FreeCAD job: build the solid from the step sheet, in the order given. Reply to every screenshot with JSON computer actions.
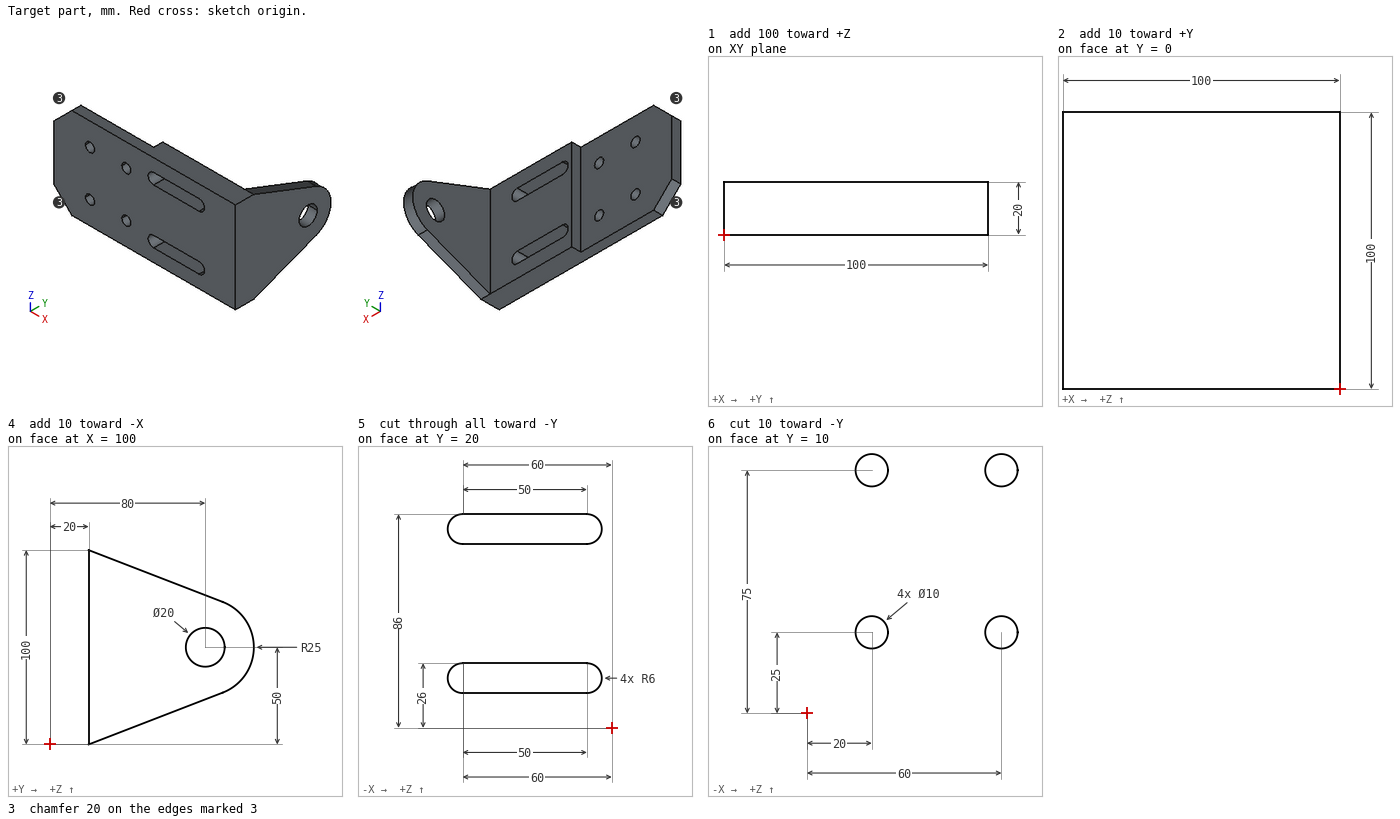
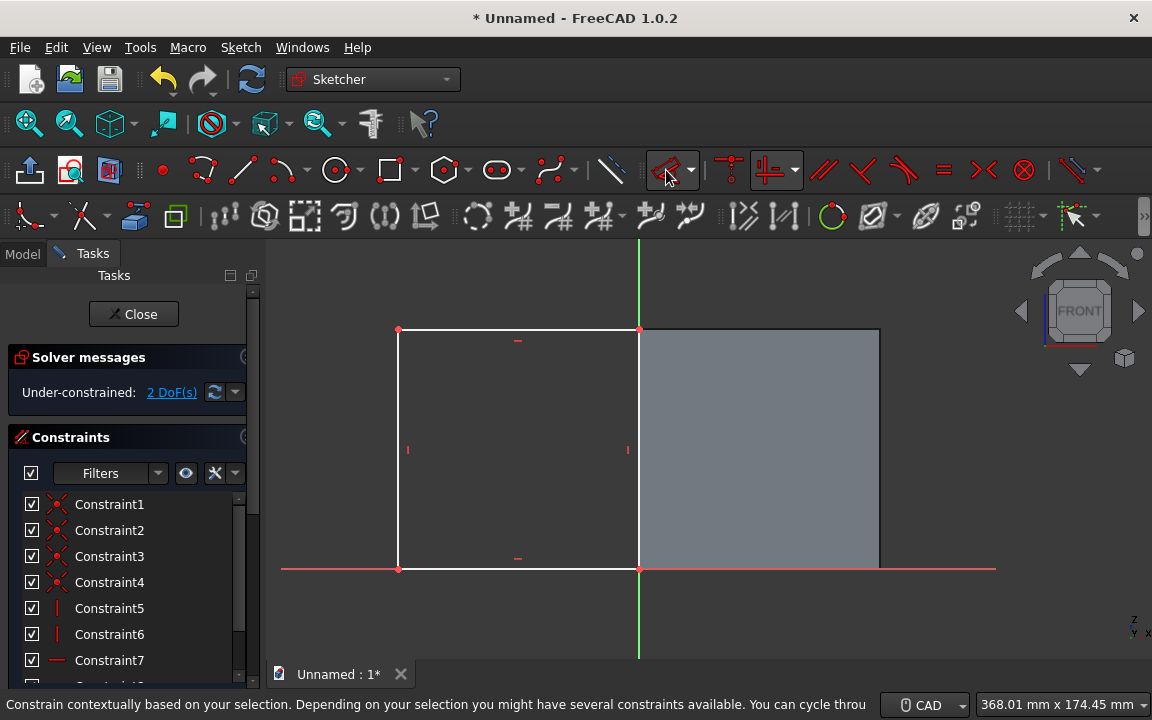
{"action": "left_click", "coordinate": [639, 498]}
{"action": "left_click", "coordinate": [673, 450]}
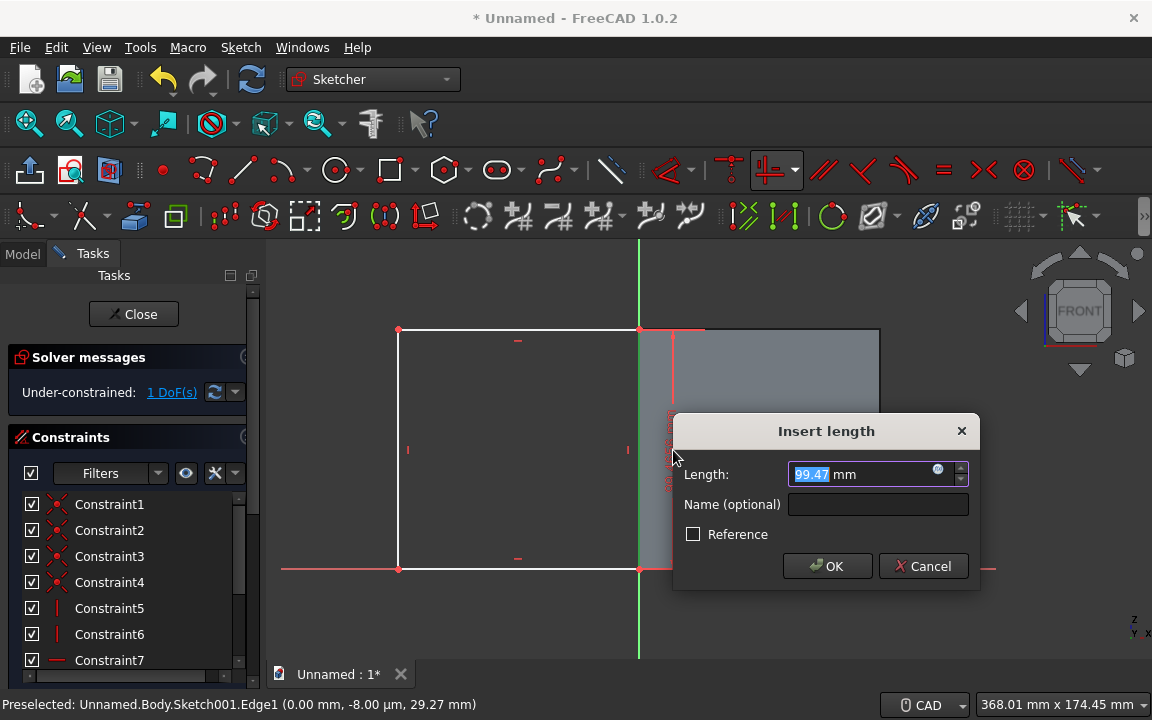
{"action": "type", "text": "100"}
{"action": "key", "text": "Return"}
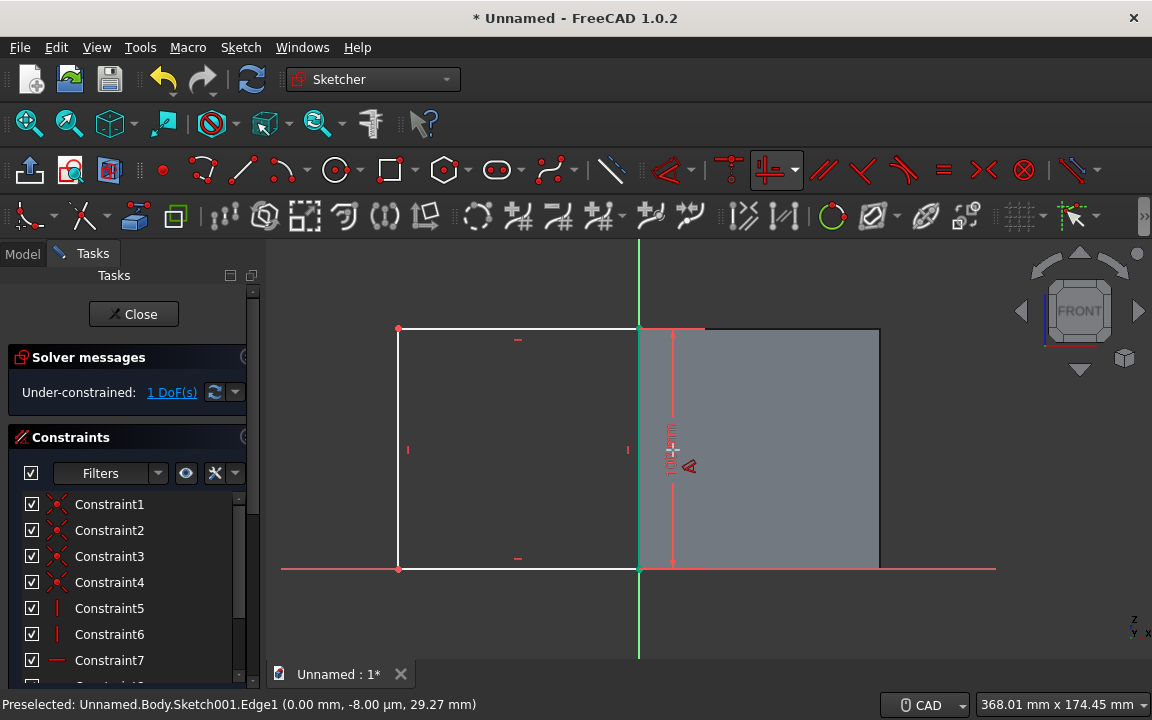
{"action": "left_click", "coordinate": [567, 329]}
{"action": "left_click", "coordinate": [519, 295]}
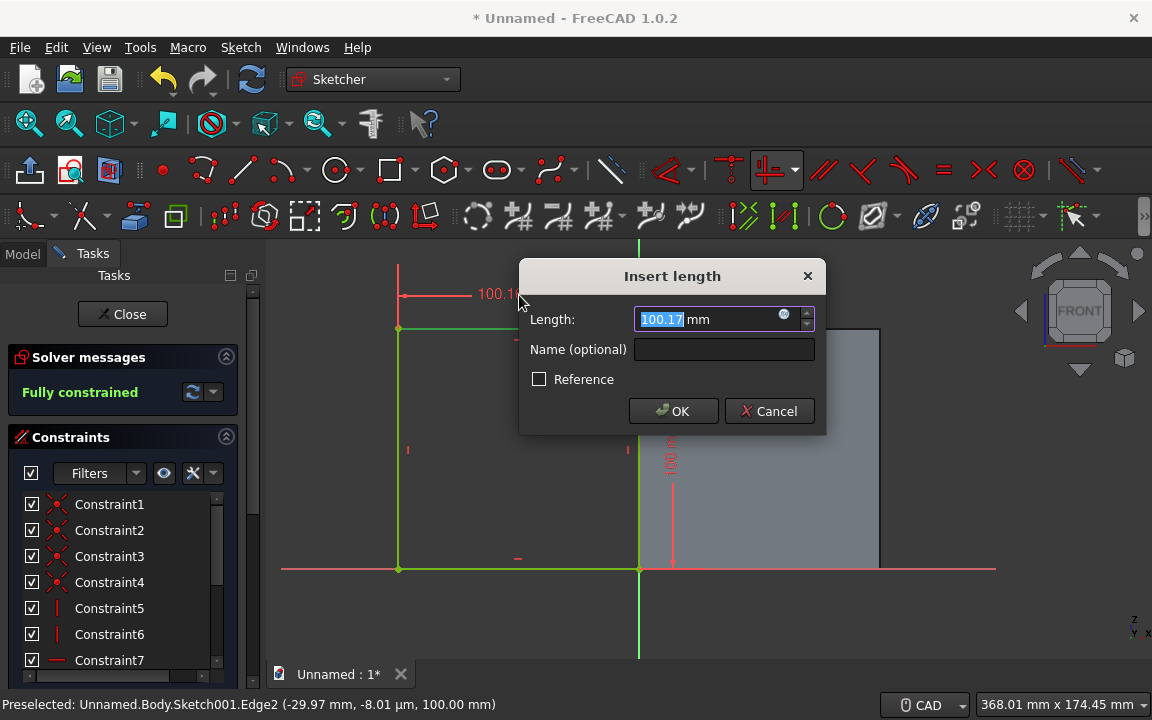
{"action": "type", "text": "100"}
{"action": "key", "text": "Return"}
{"action": "key", "text": "Escape"}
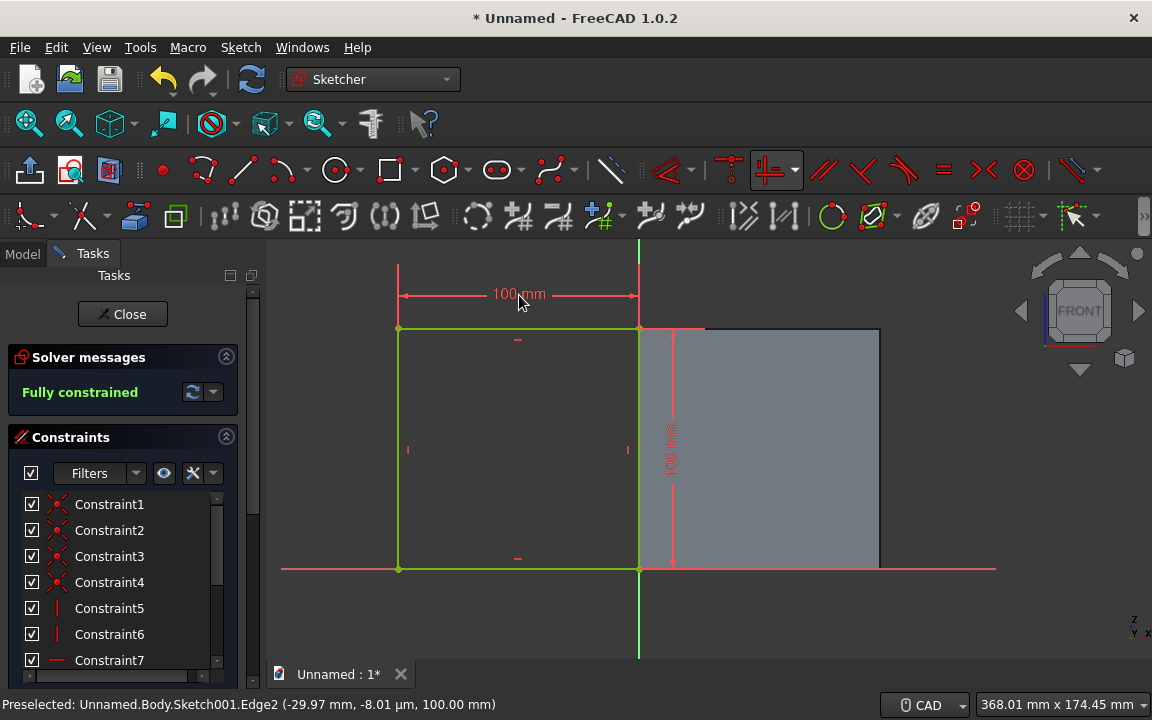
{"action": "left_click", "coordinate": [123, 314]}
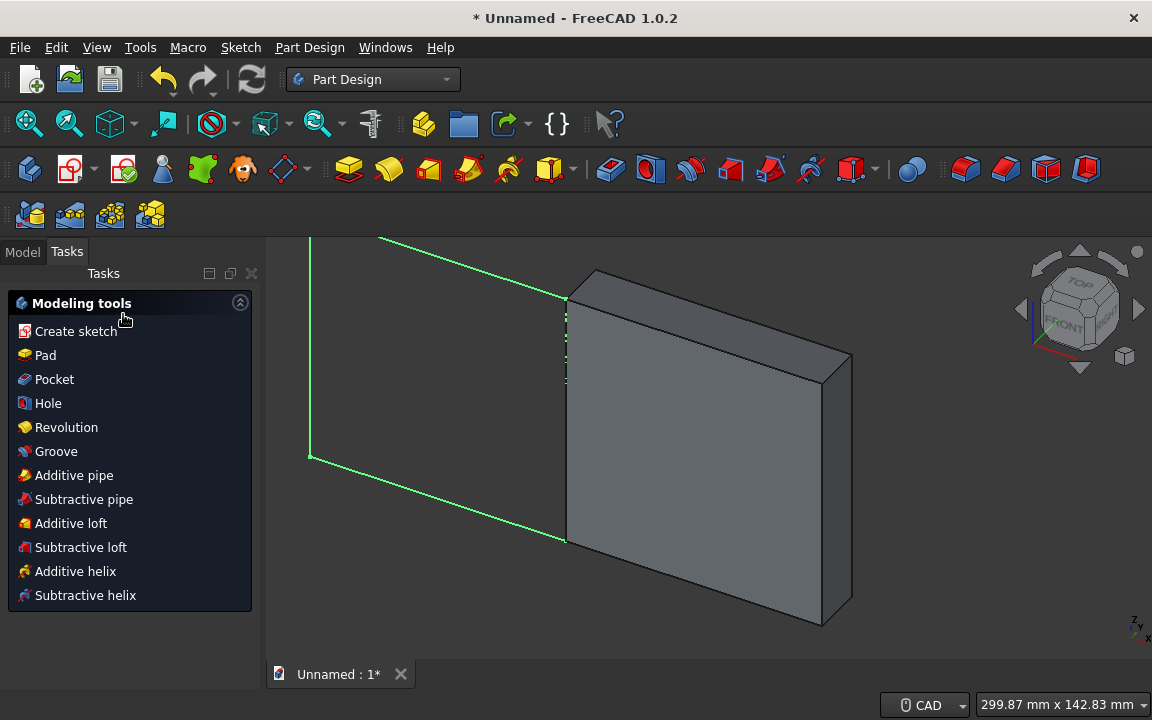
{"action": "left_click", "coordinate": [350, 170]}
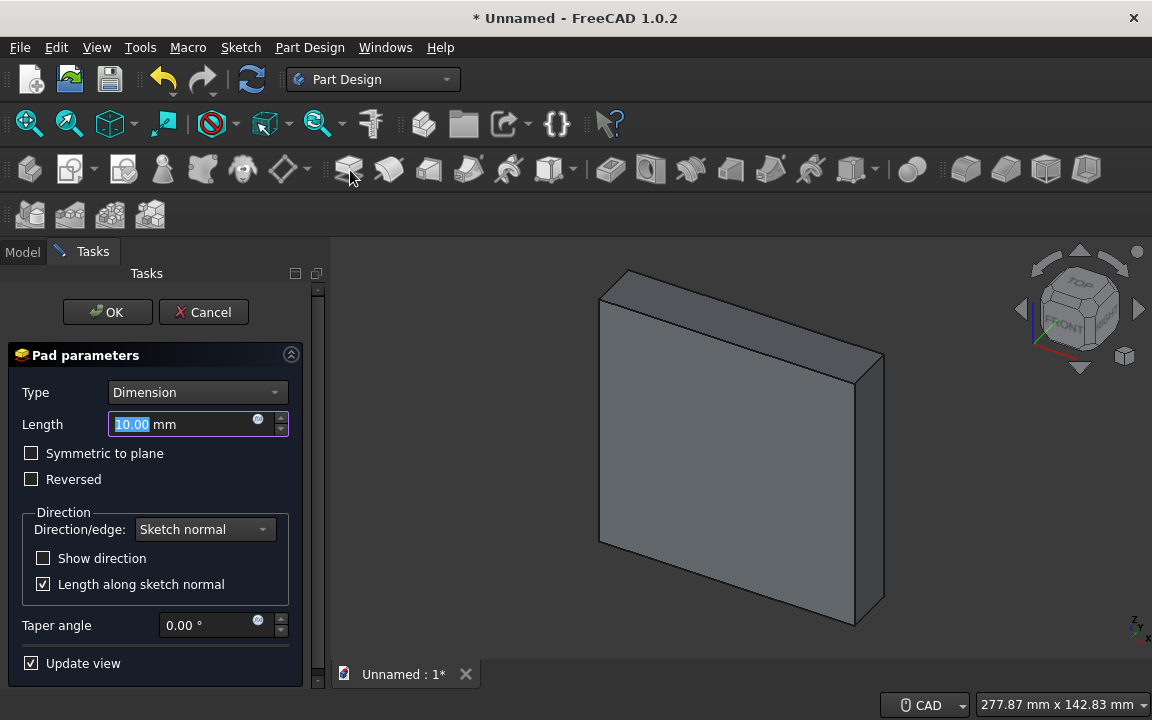
{"action": "type", "text": "10"}
{"action": "key", "text": "Tab"}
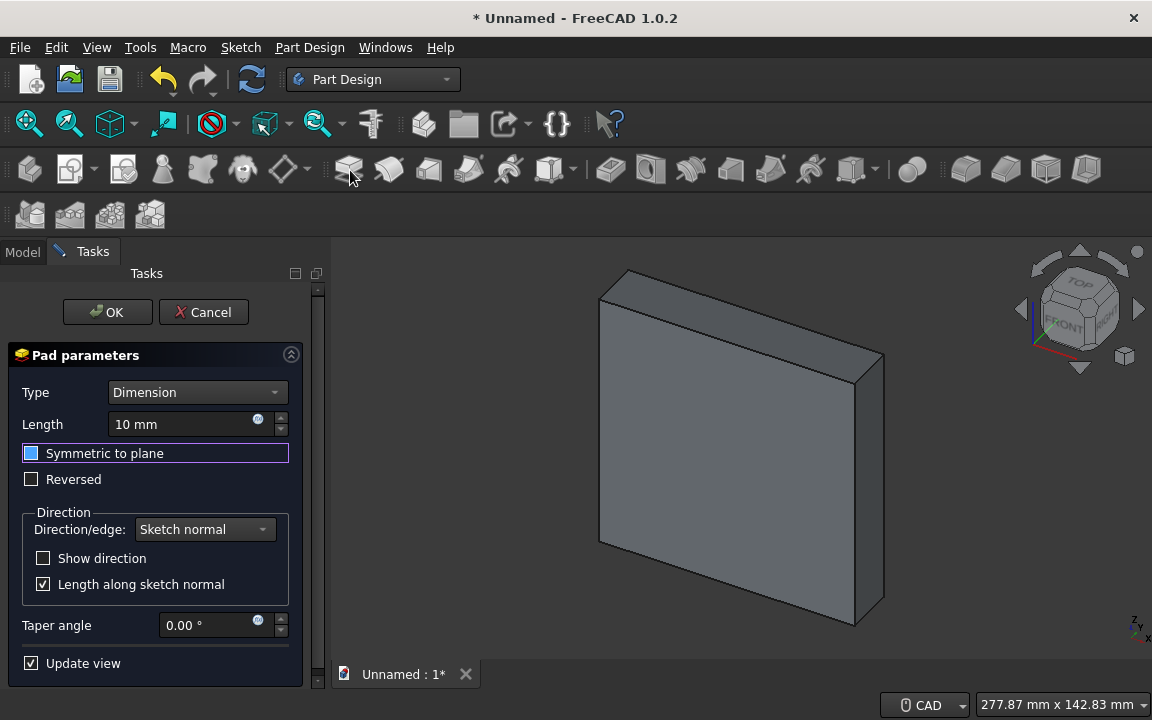
{"action": "left_click", "coordinate": [30, 479]}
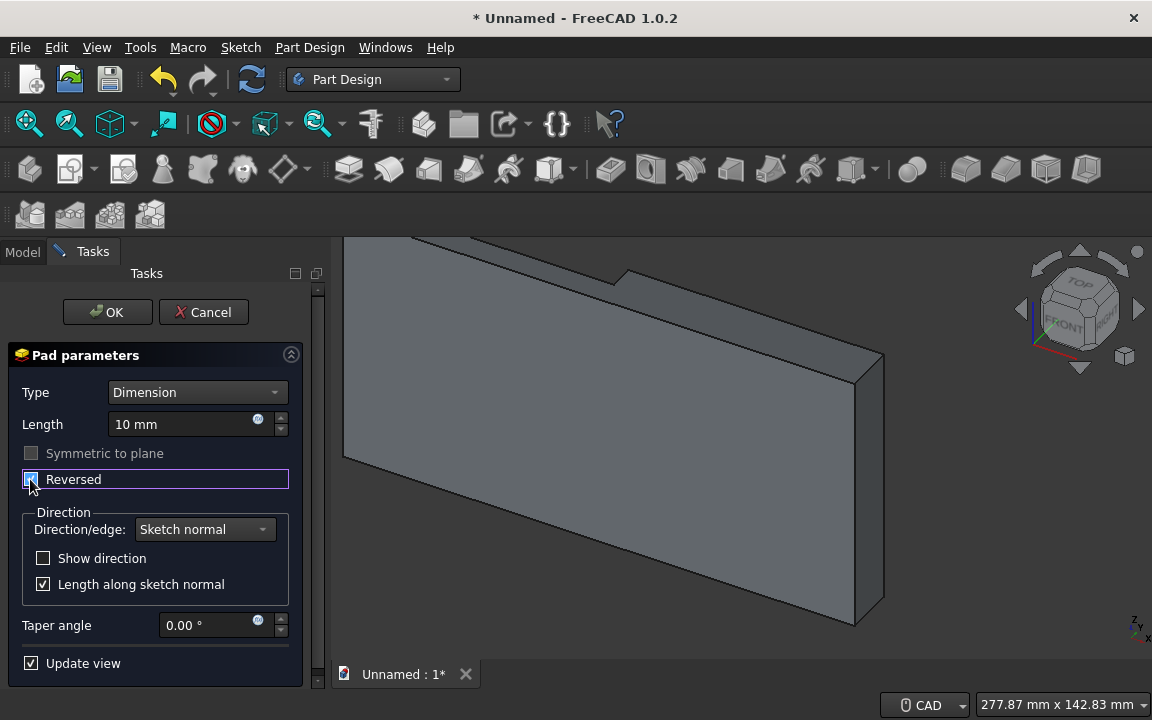
{"action": "left_click", "coordinate": [108, 312]}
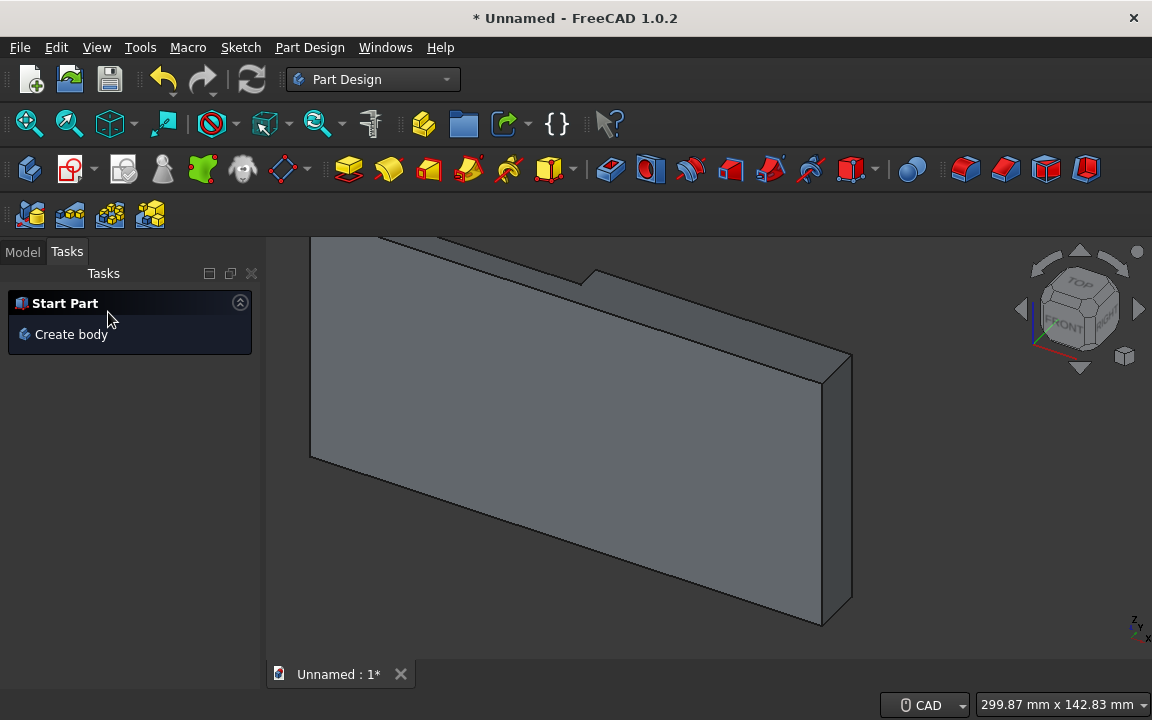
{"action": "left_click", "coordinate": [30, 124]}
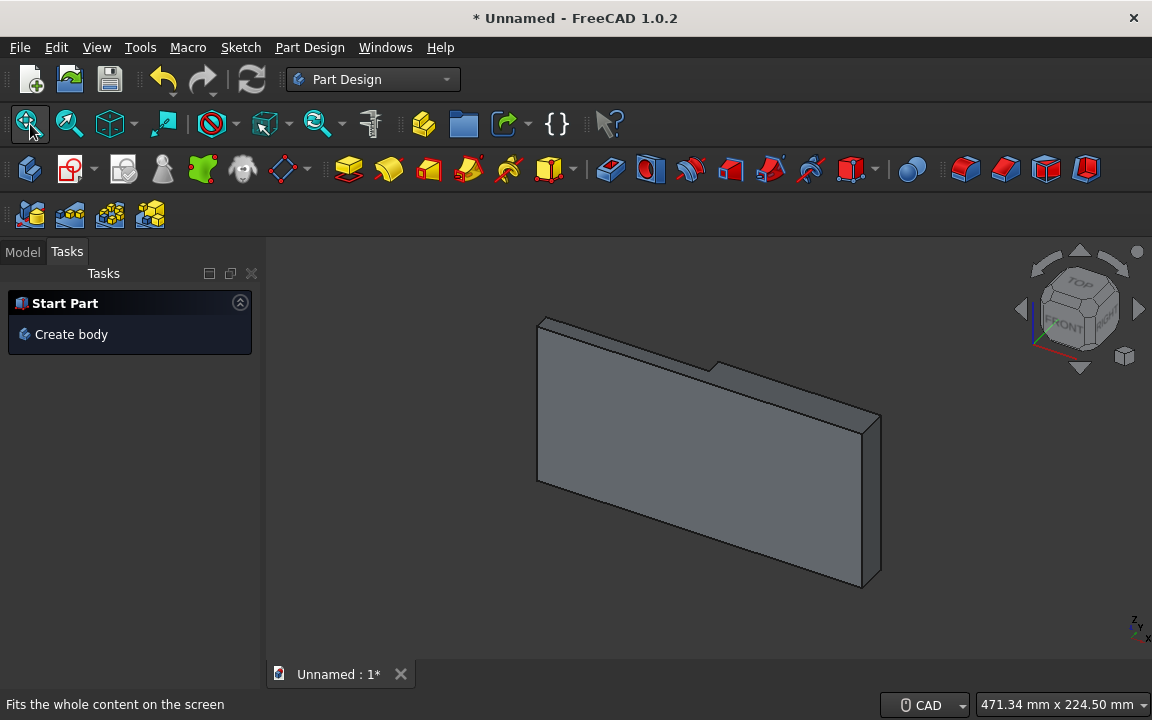
{"action": "scroll", "coordinate": [542, 475], "scroll_direction": "up", "scroll_amount": 4}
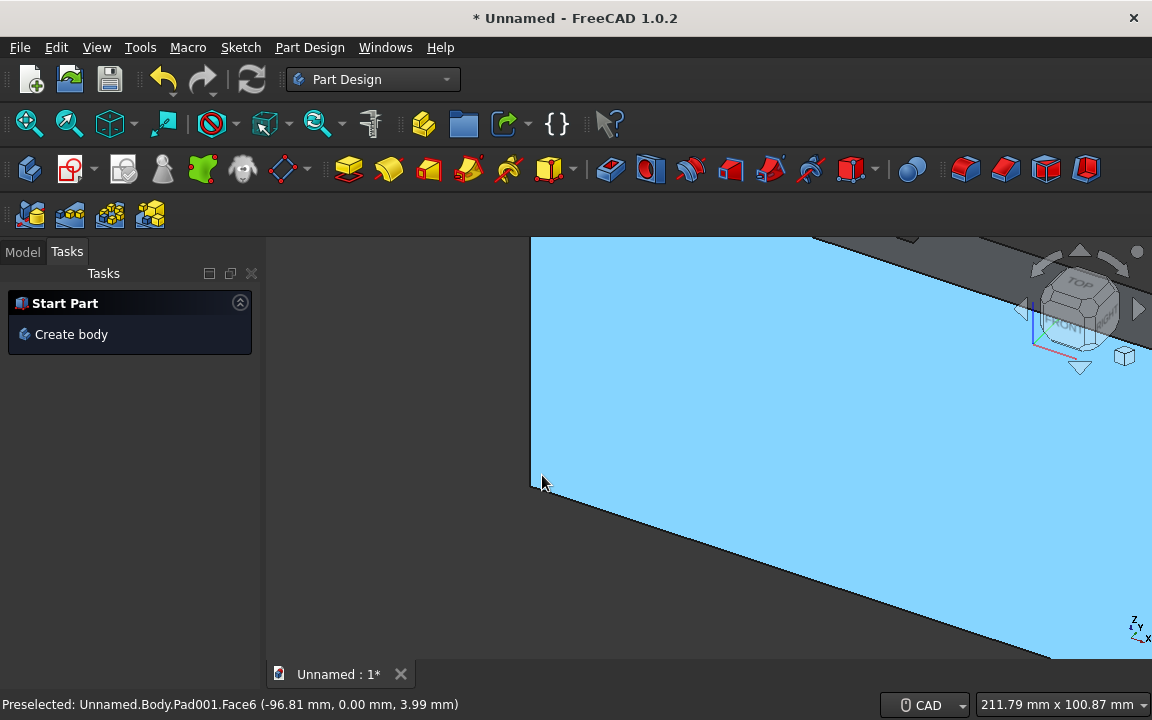
{"action": "left_click", "coordinate": [30, 124]}